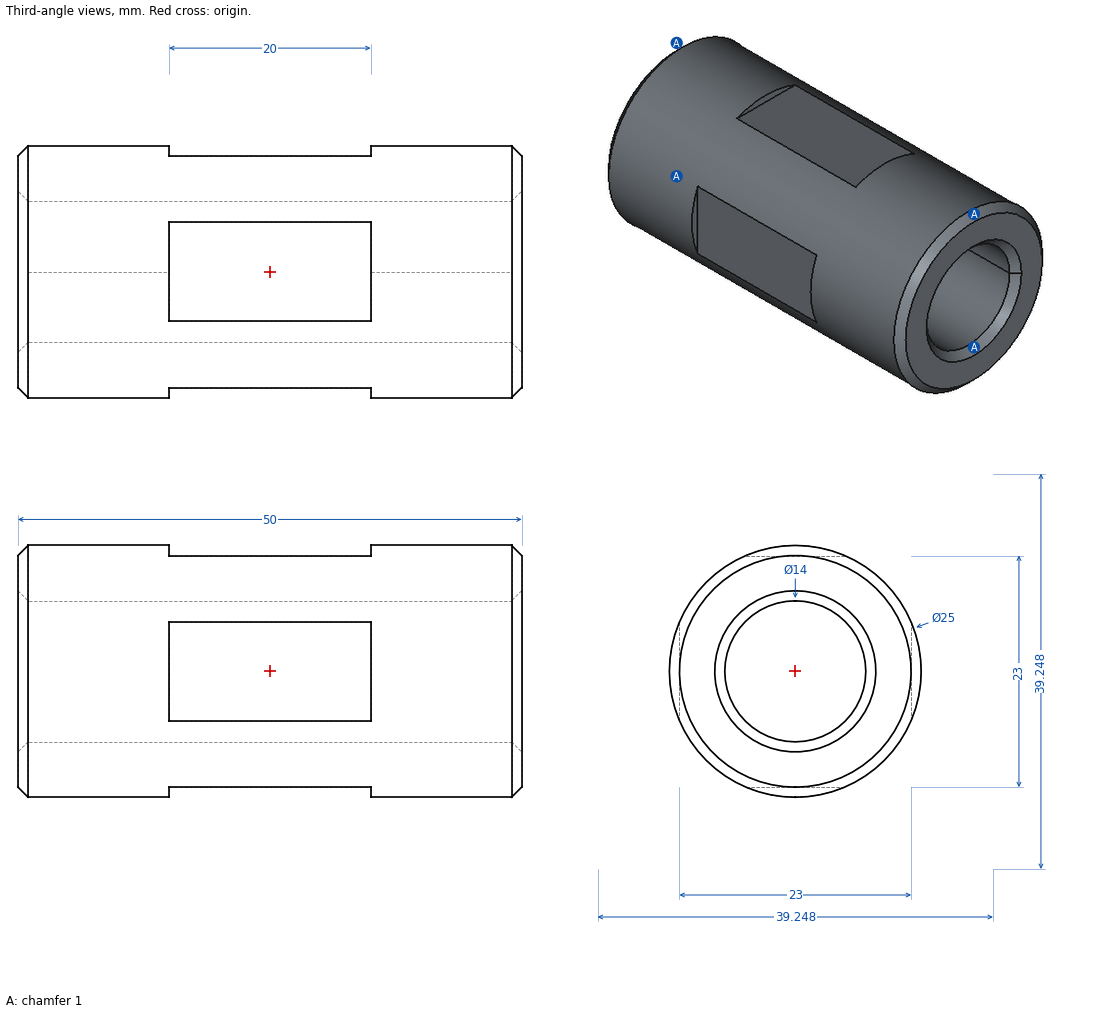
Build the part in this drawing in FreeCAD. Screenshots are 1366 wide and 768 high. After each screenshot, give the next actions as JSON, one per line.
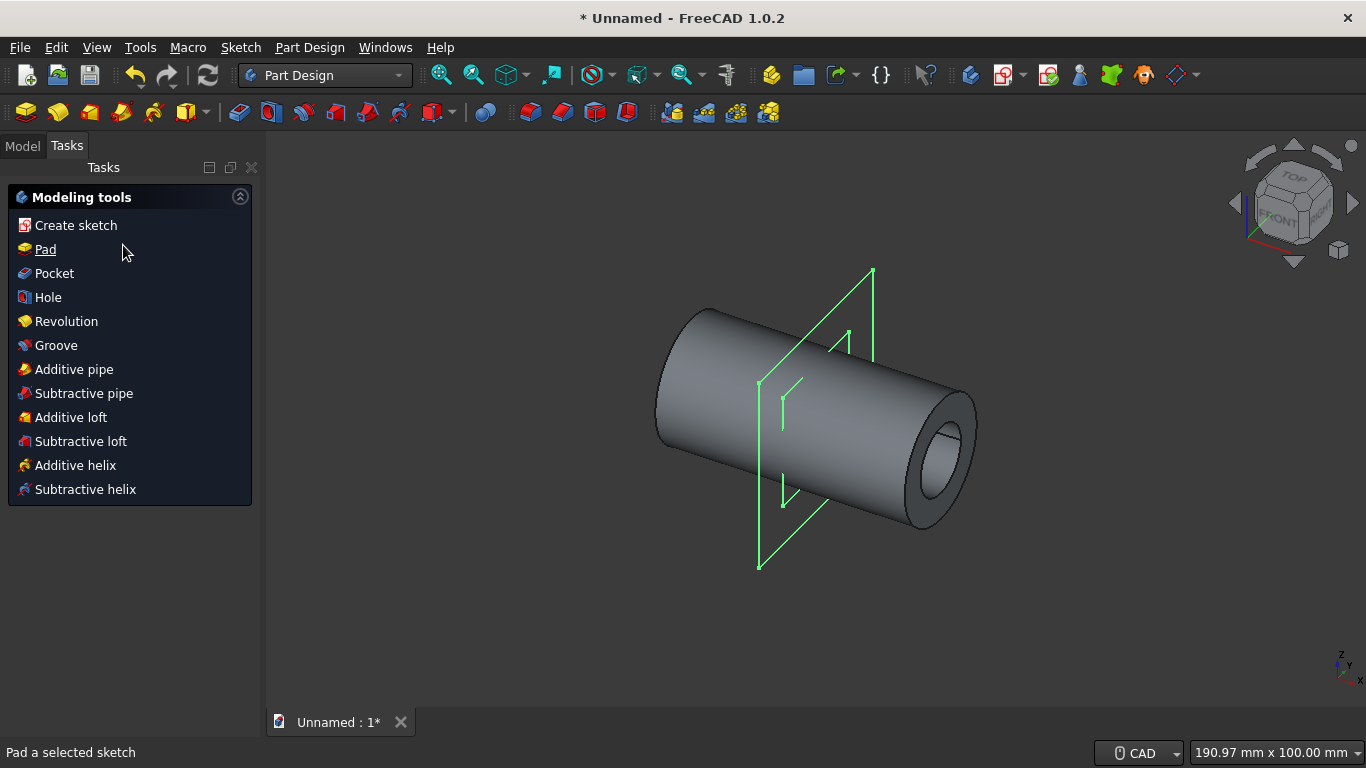
{"action": "left_click", "coordinate": [240, 112]}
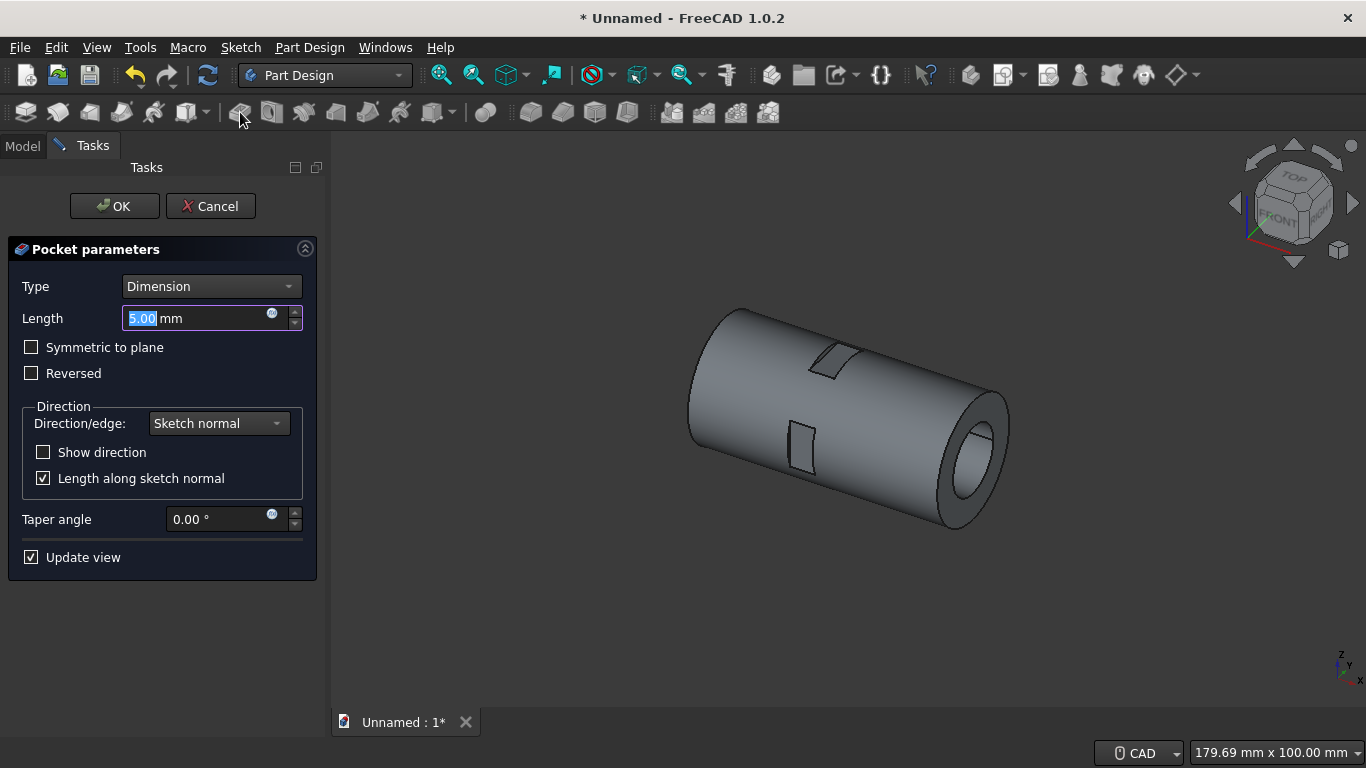
{"action": "type", "text": "20"}
{"action": "key", "text": "Tab"}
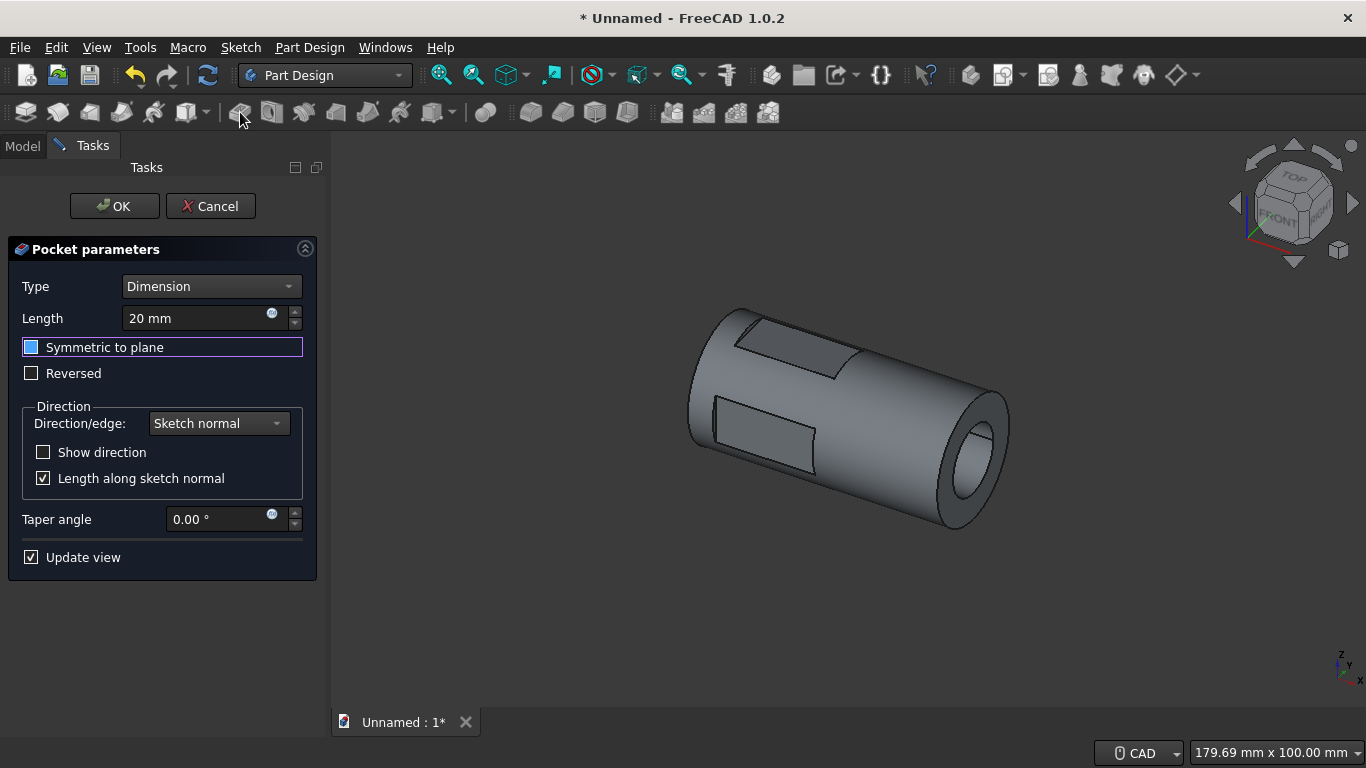
{"action": "left_click", "coordinate": [30, 347]}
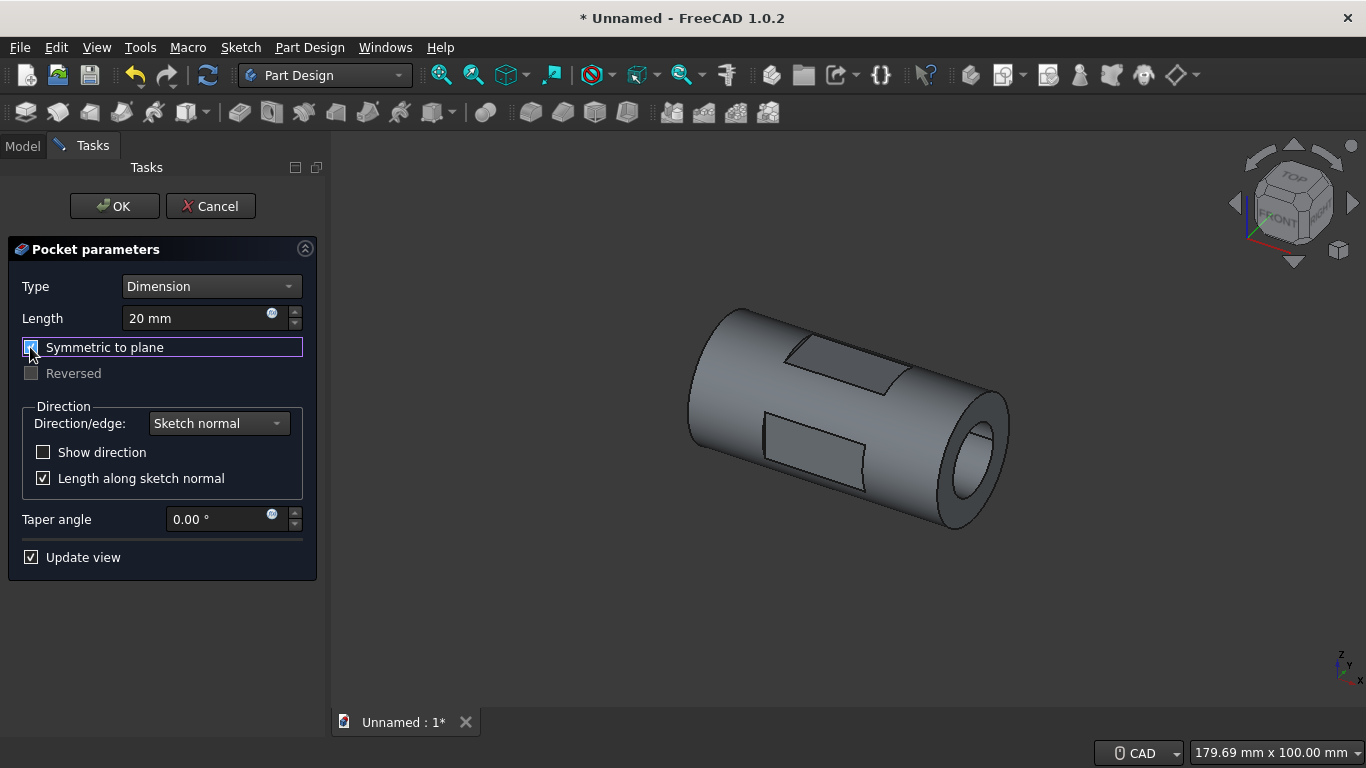
{"action": "left_click", "coordinate": [115, 206]}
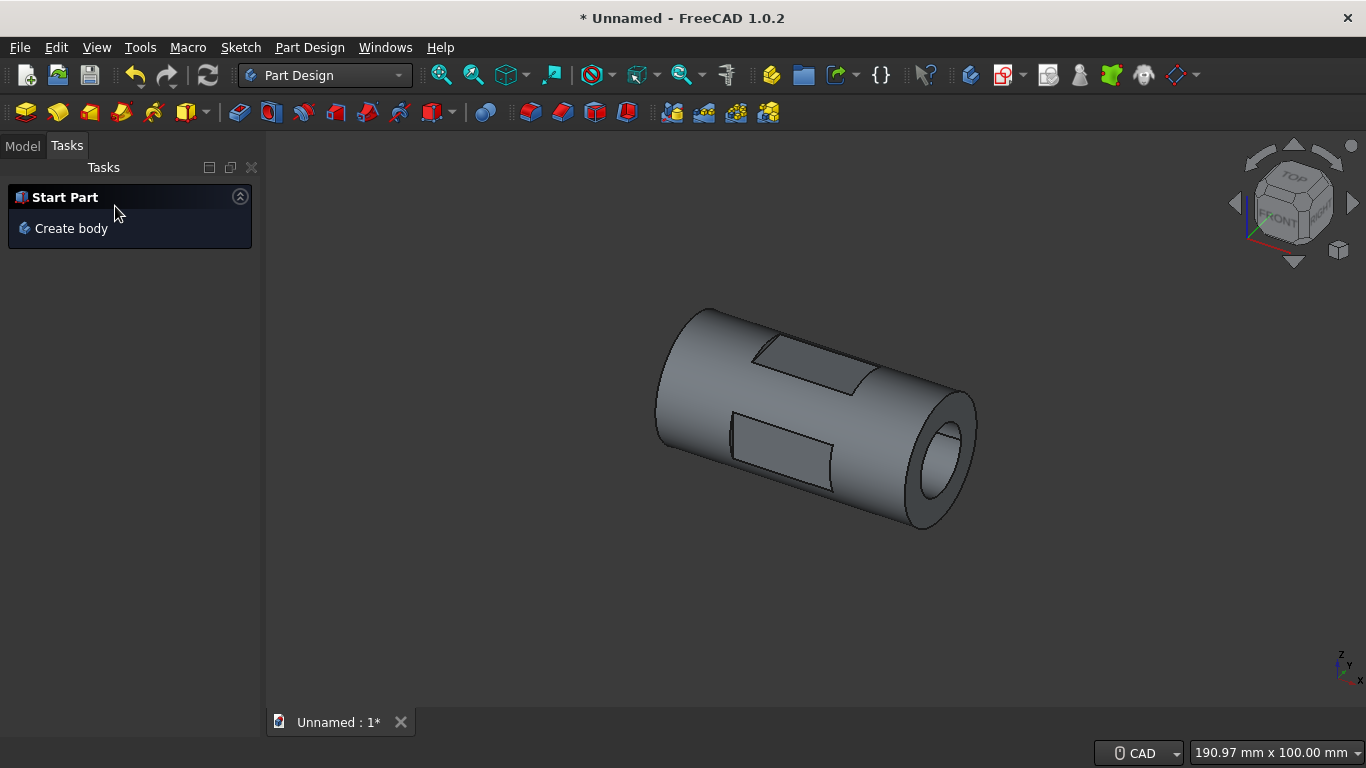
{"action": "left_click", "coordinate": [905, 495]}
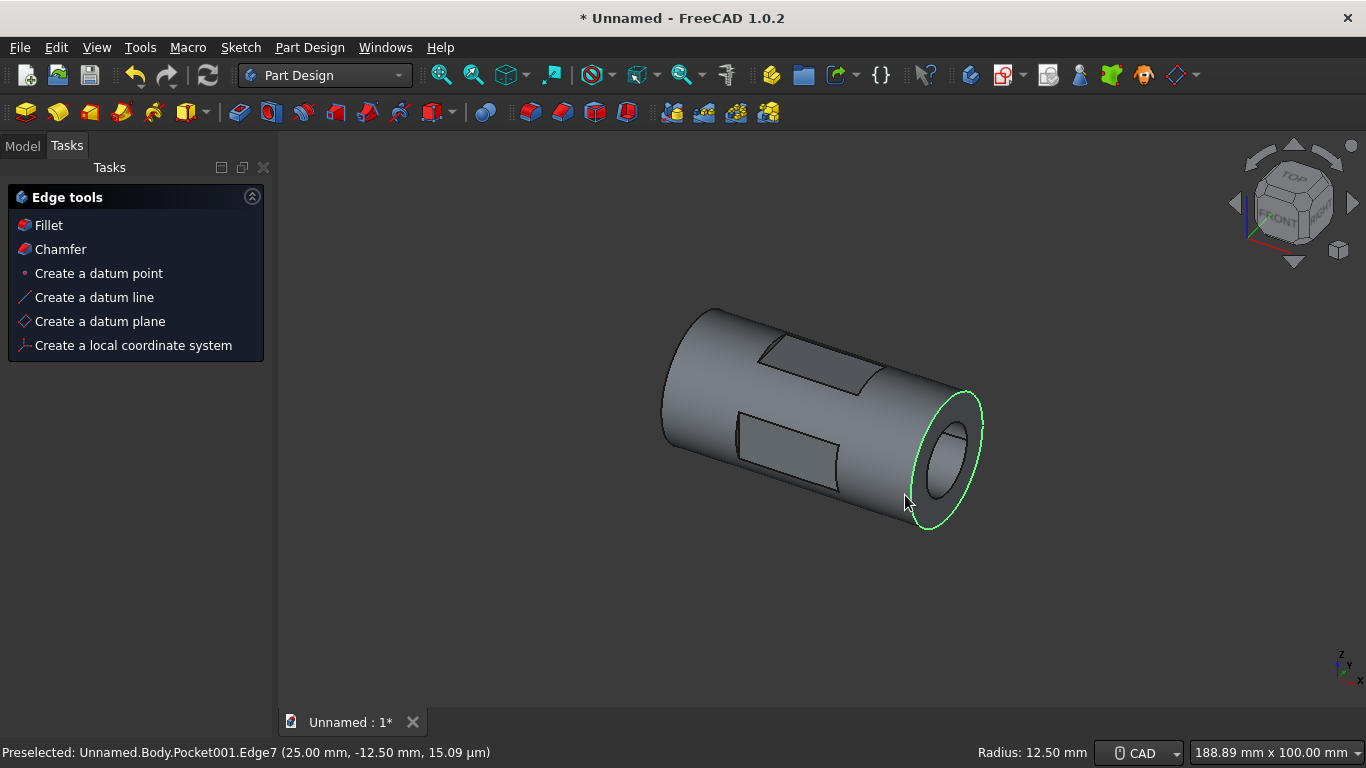
{"action": "left_click", "coordinate": [940, 497], "text": "ctrl"}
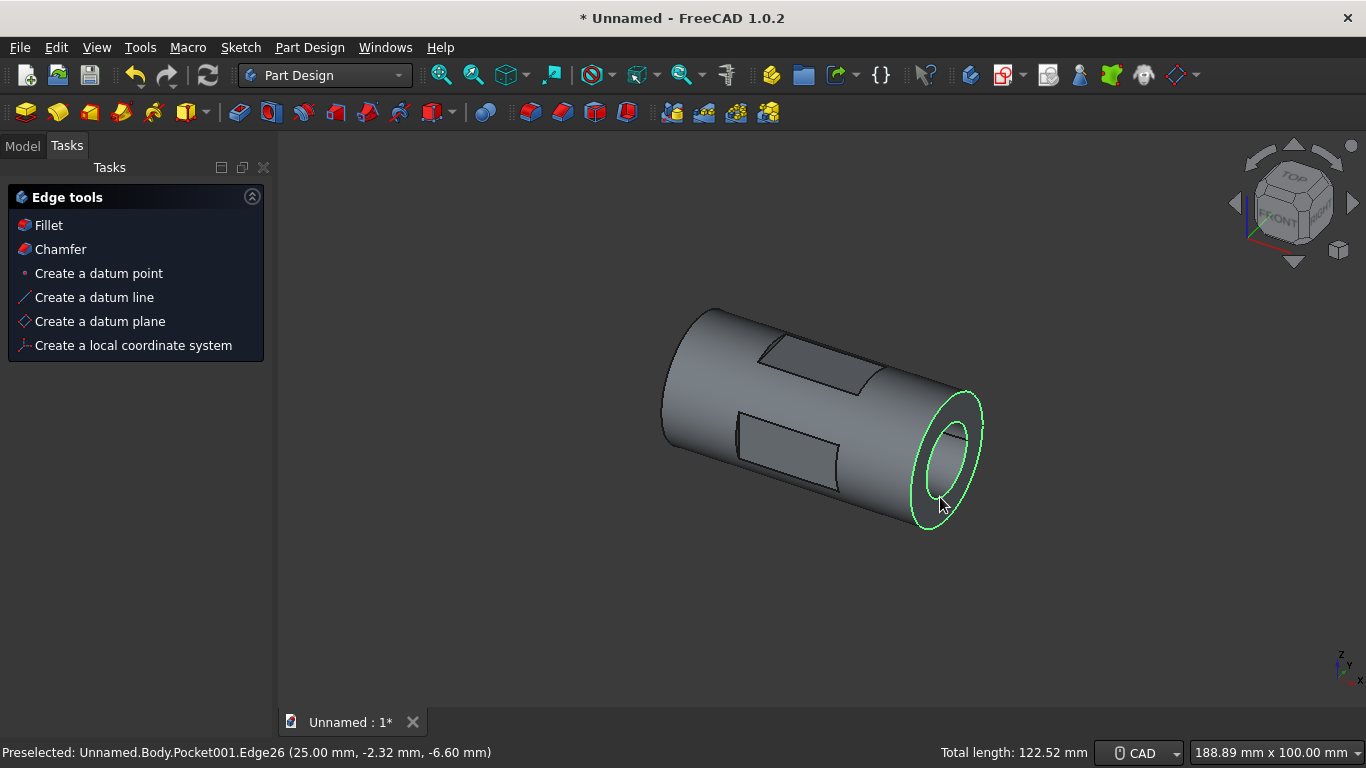
{"action": "key", "text": "0"}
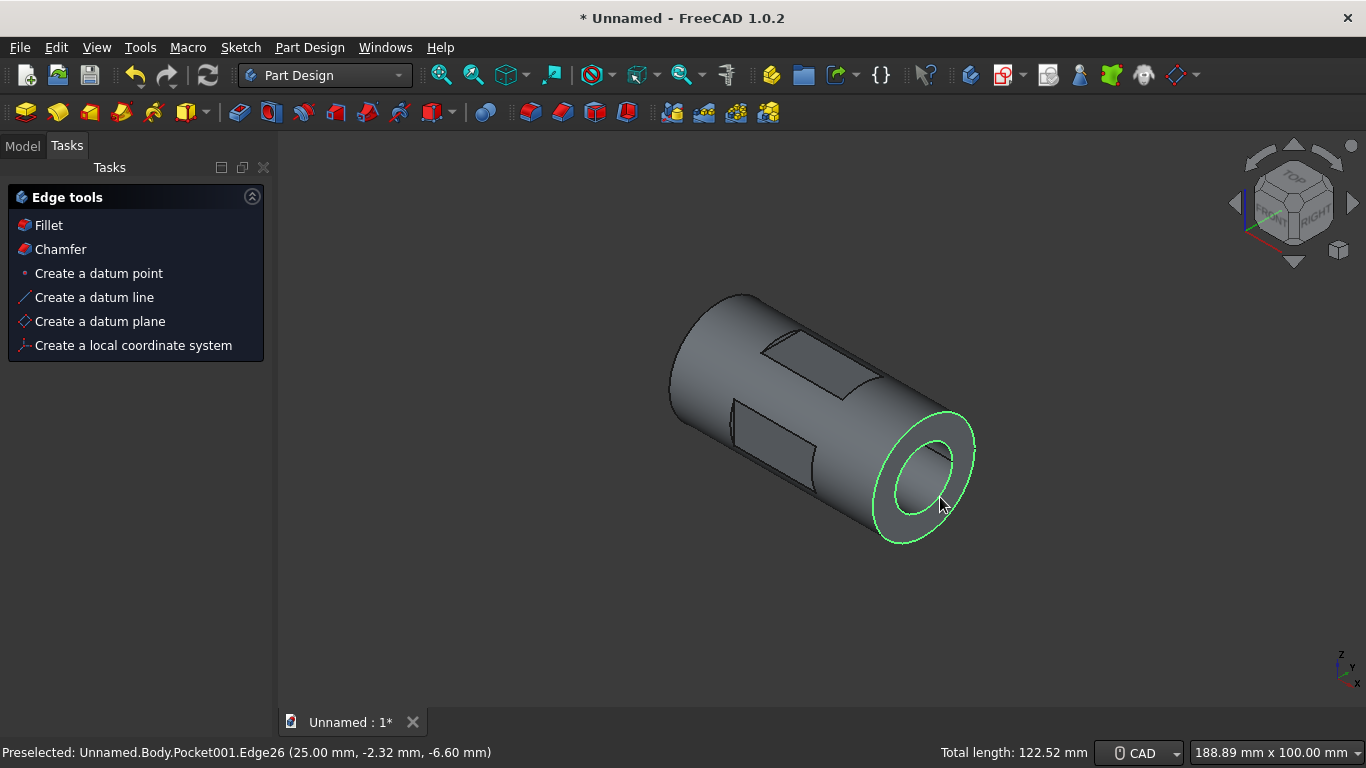
{"action": "key", "text": "2"}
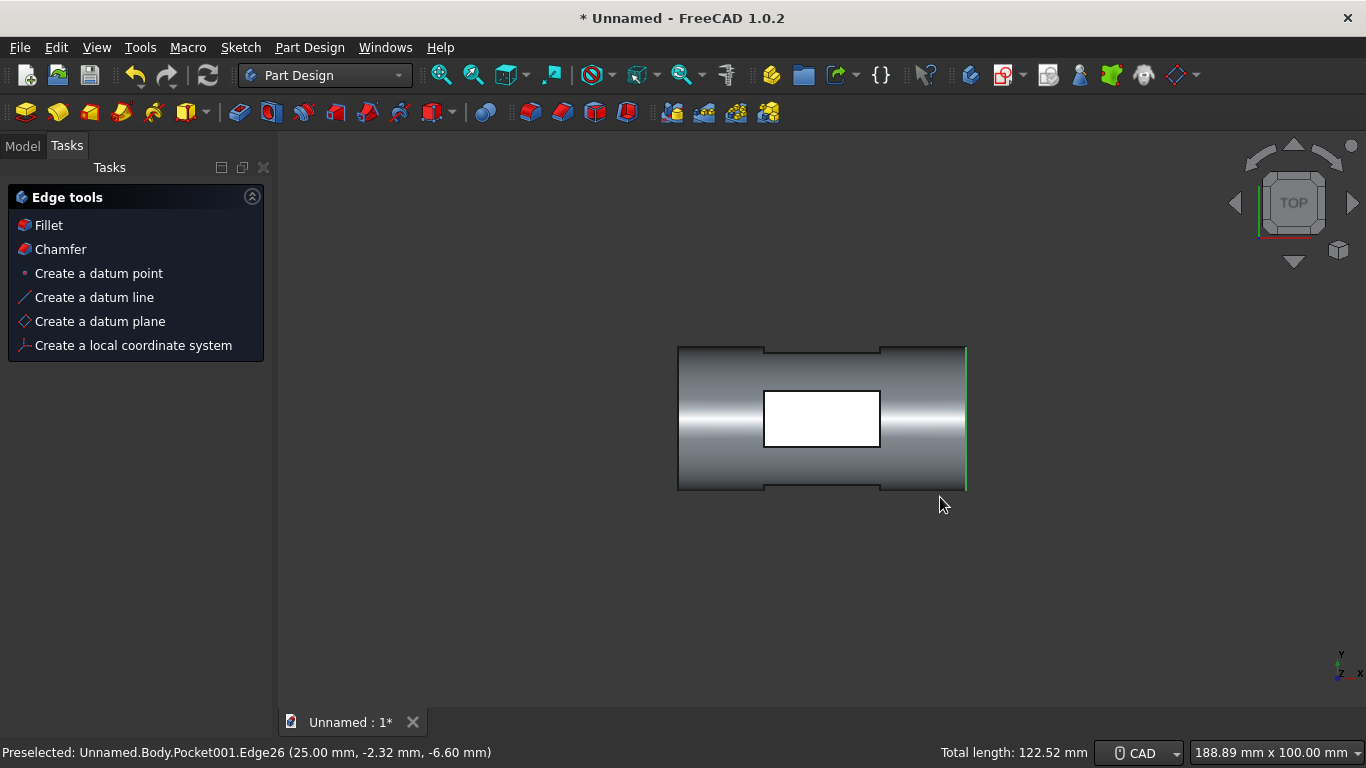
{"action": "key", "text": "v f"}